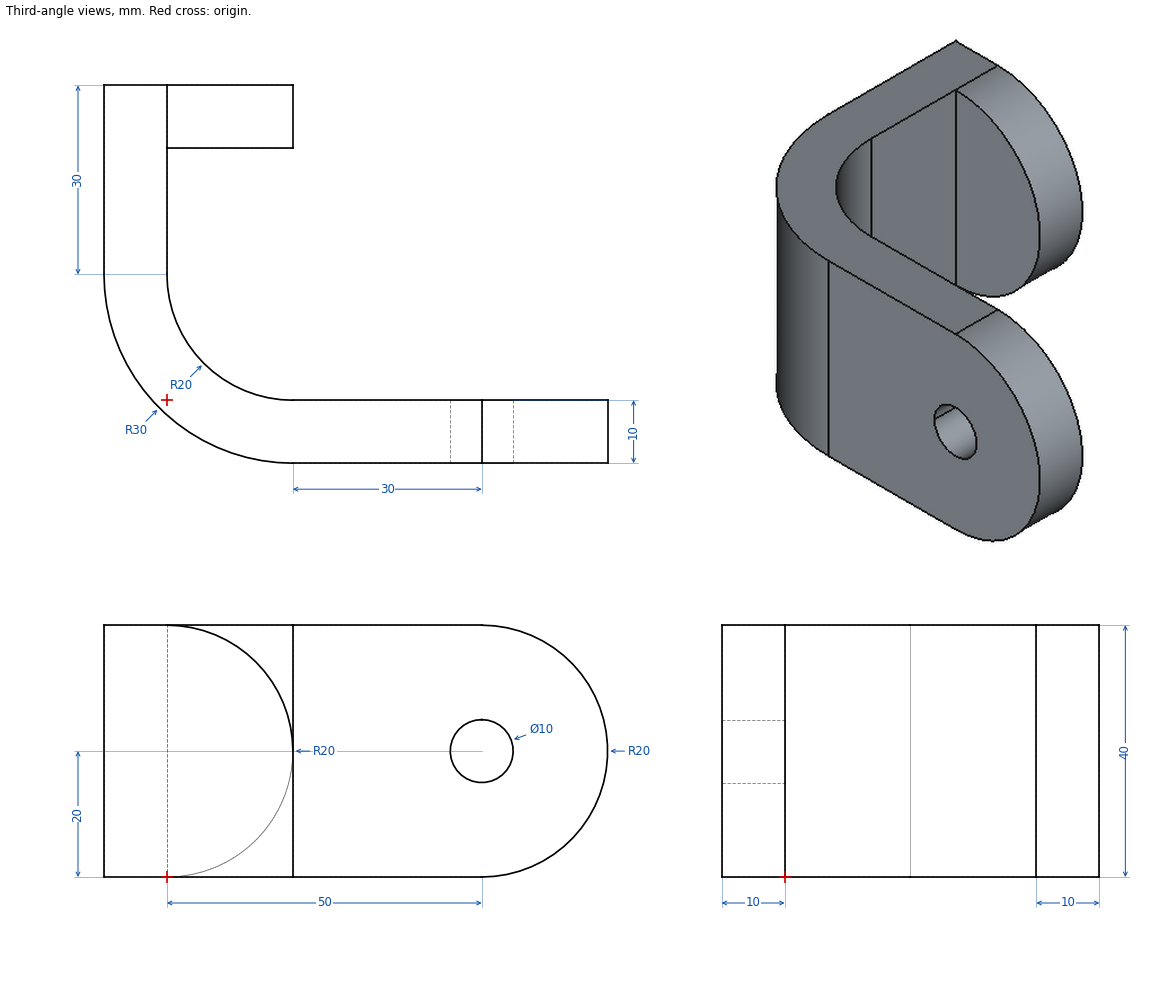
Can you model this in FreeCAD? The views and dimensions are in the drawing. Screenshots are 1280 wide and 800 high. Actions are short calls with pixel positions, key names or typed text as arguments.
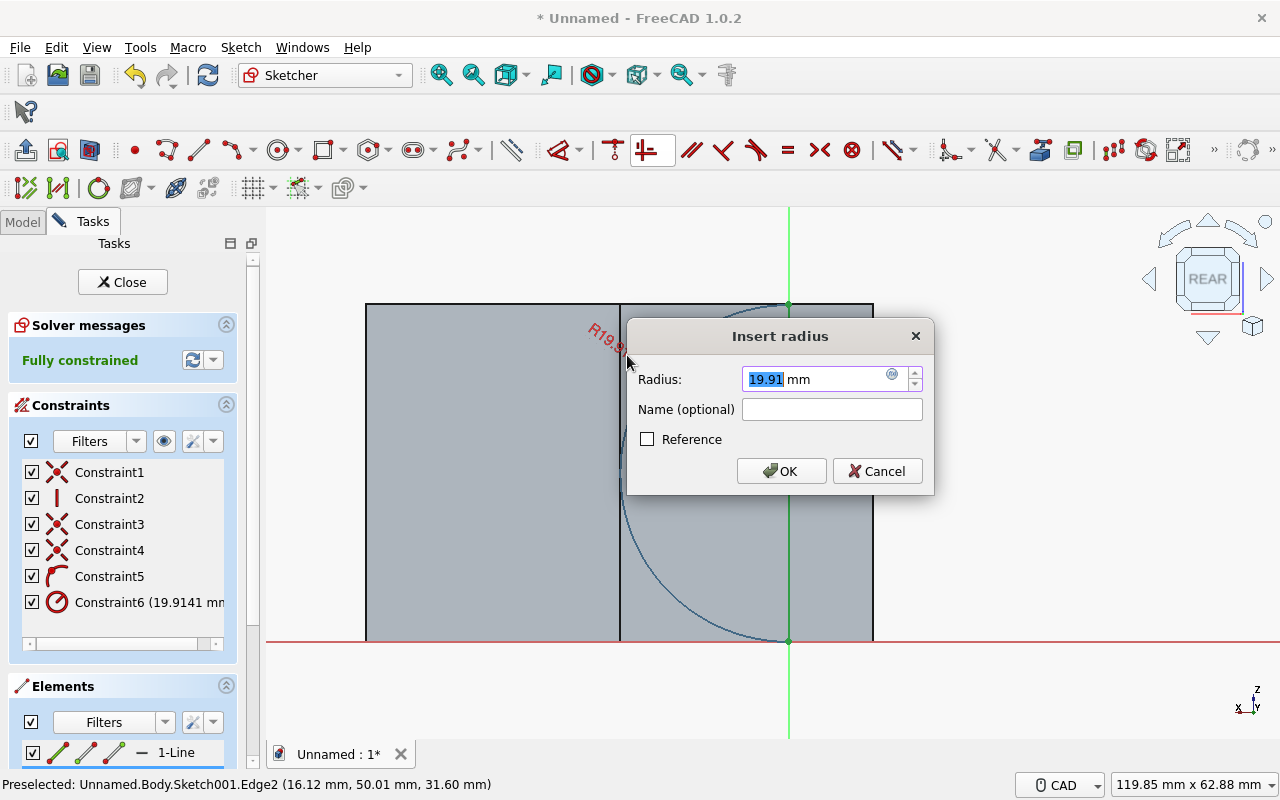
text(20)
key(Return)
key(Escape)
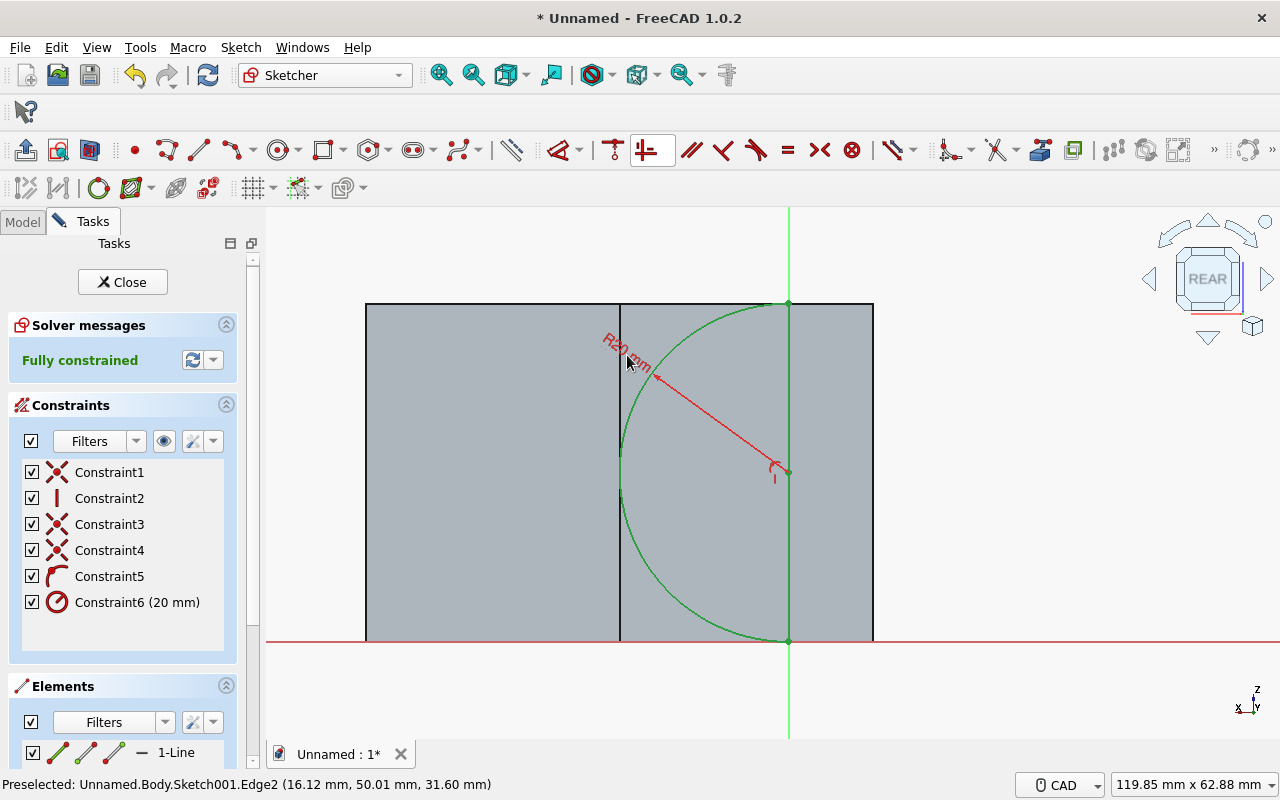
click(123, 282)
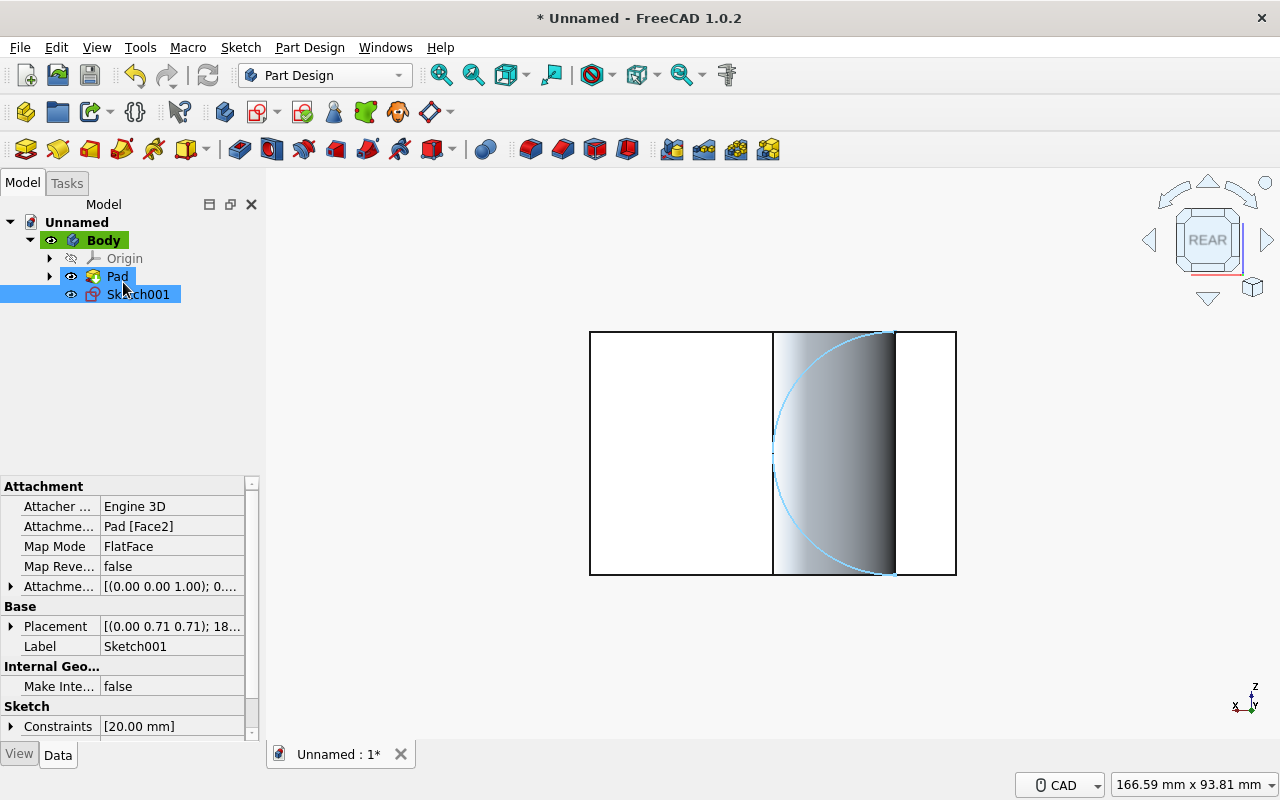
click(26, 150)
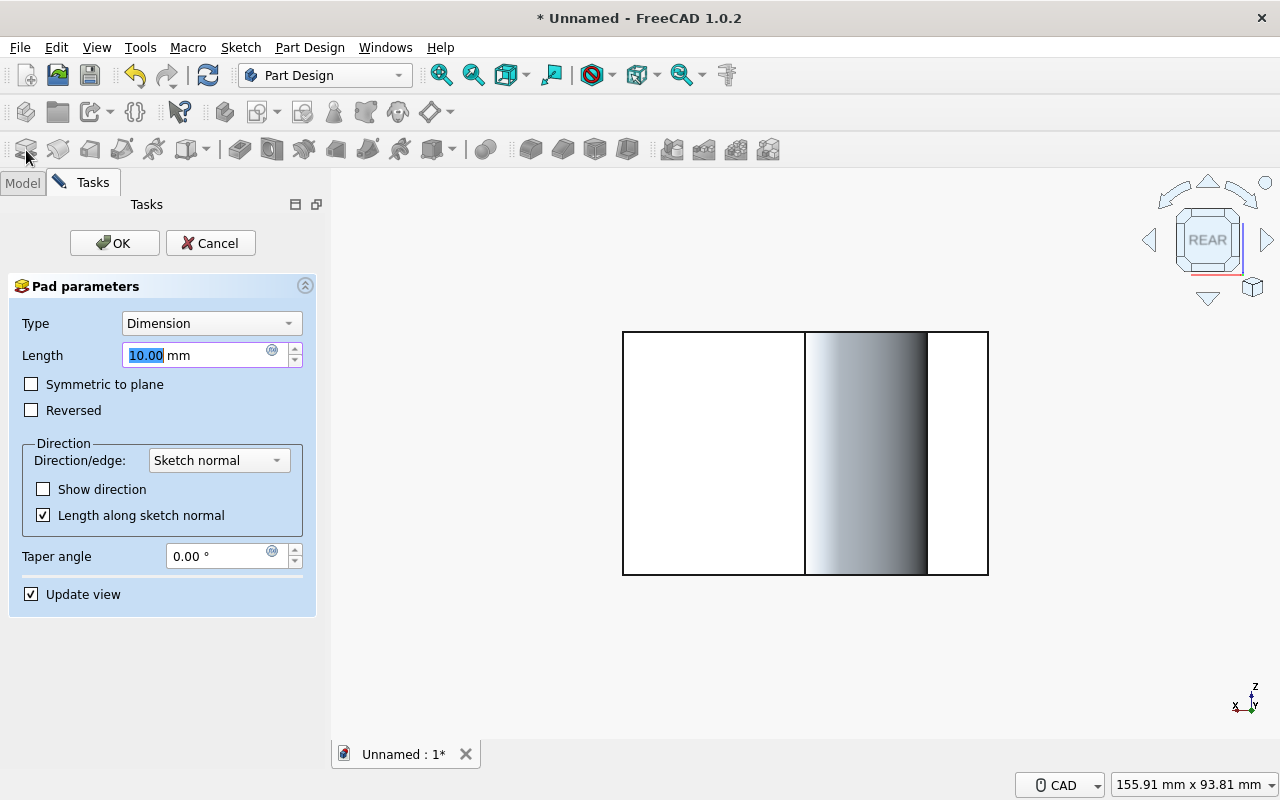
text(10)
key(Tab)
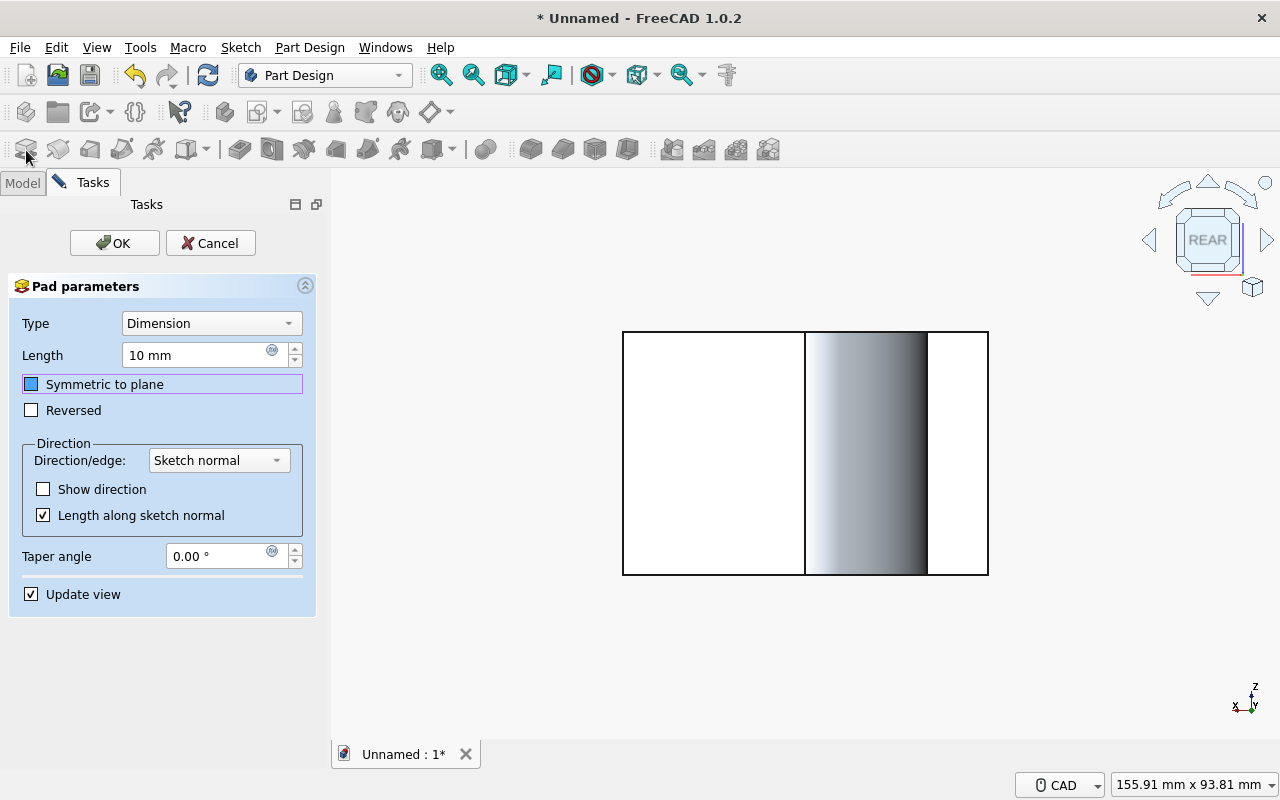
click(30, 410)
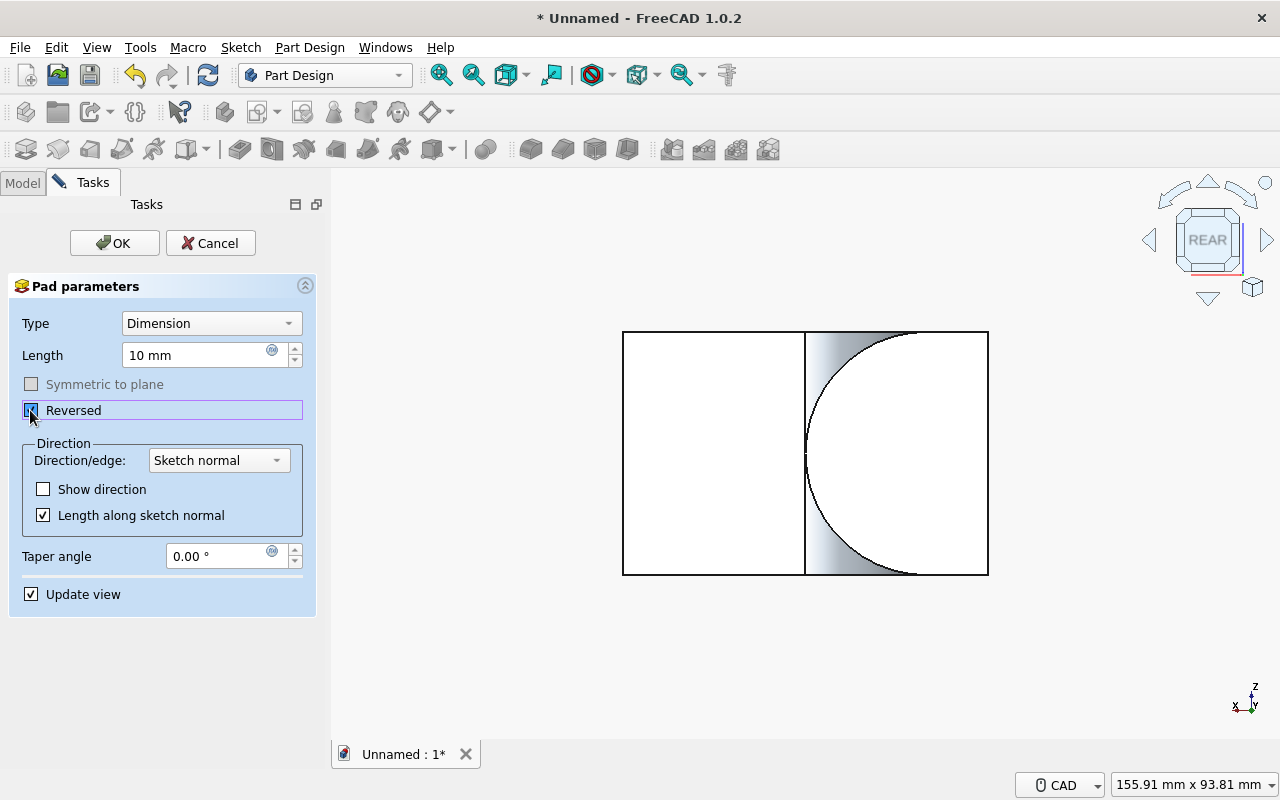
click(115, 243)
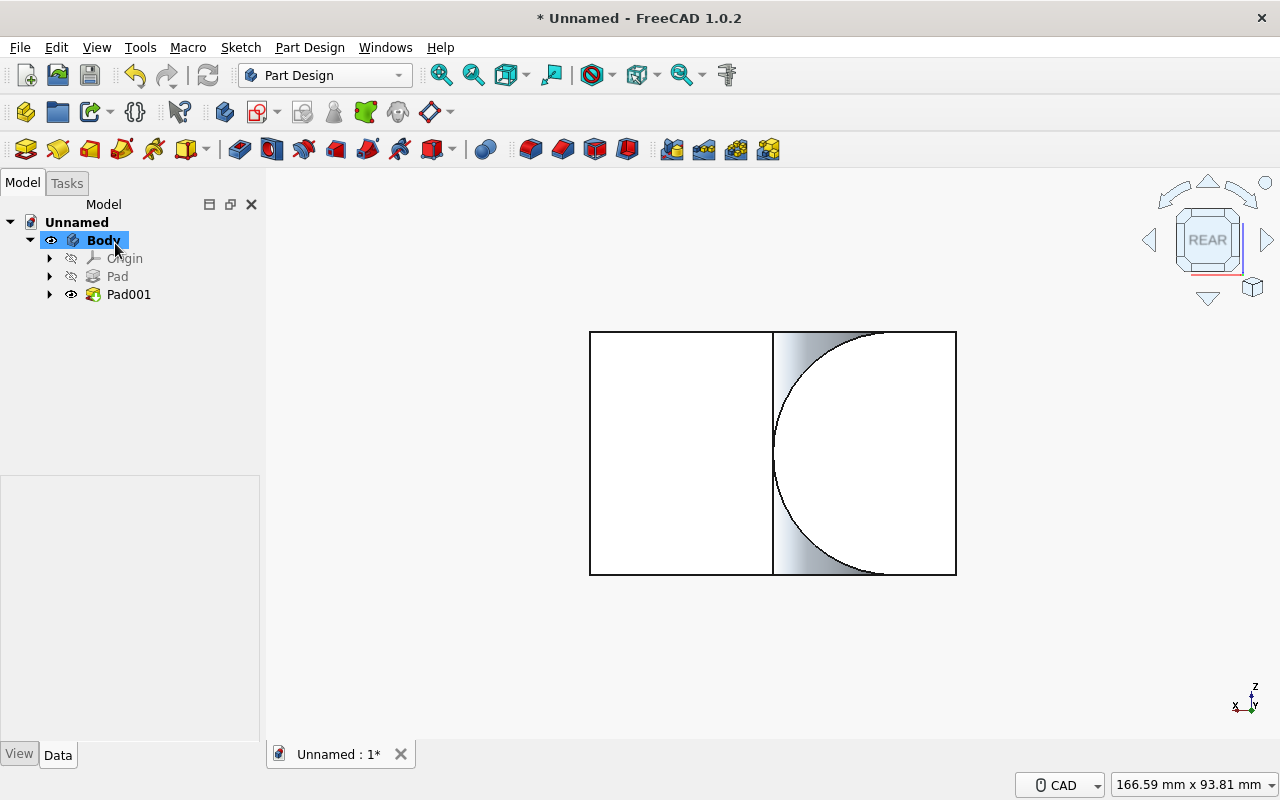
click(442, 76)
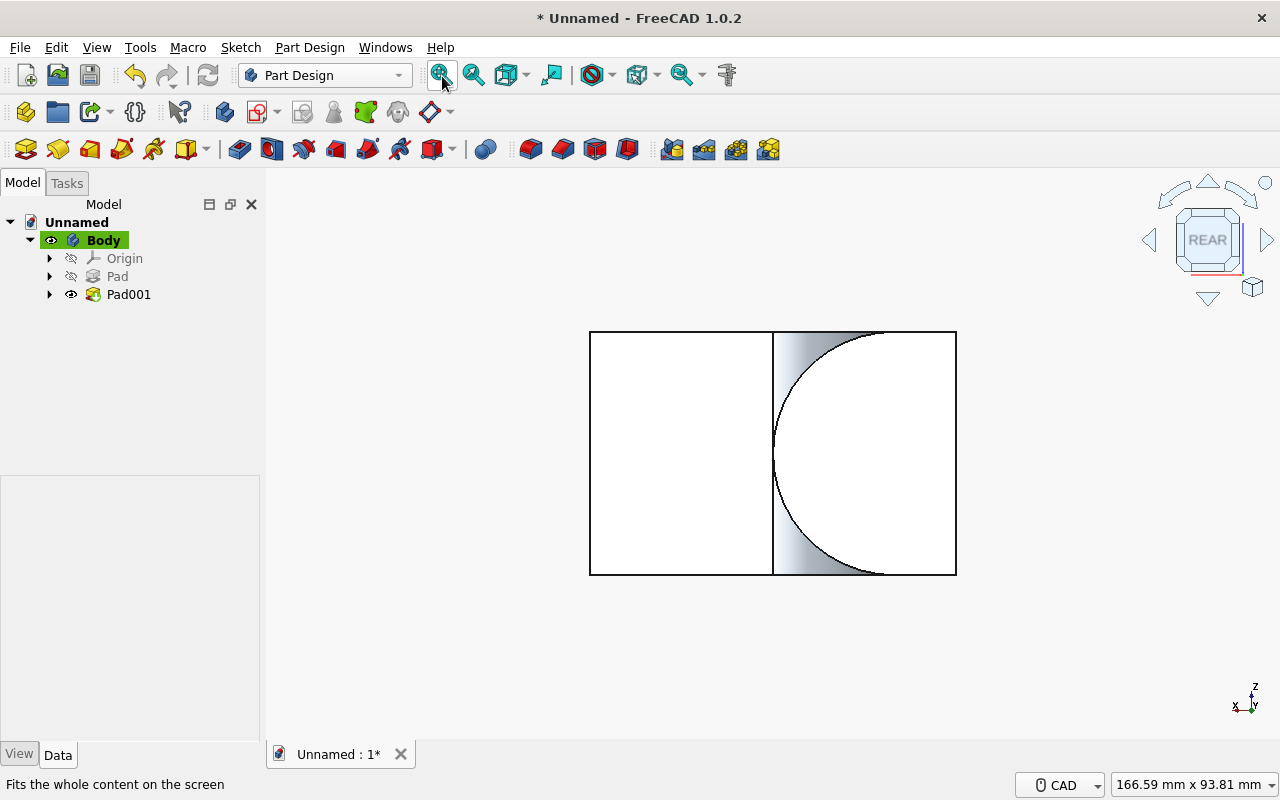
click(682, 452)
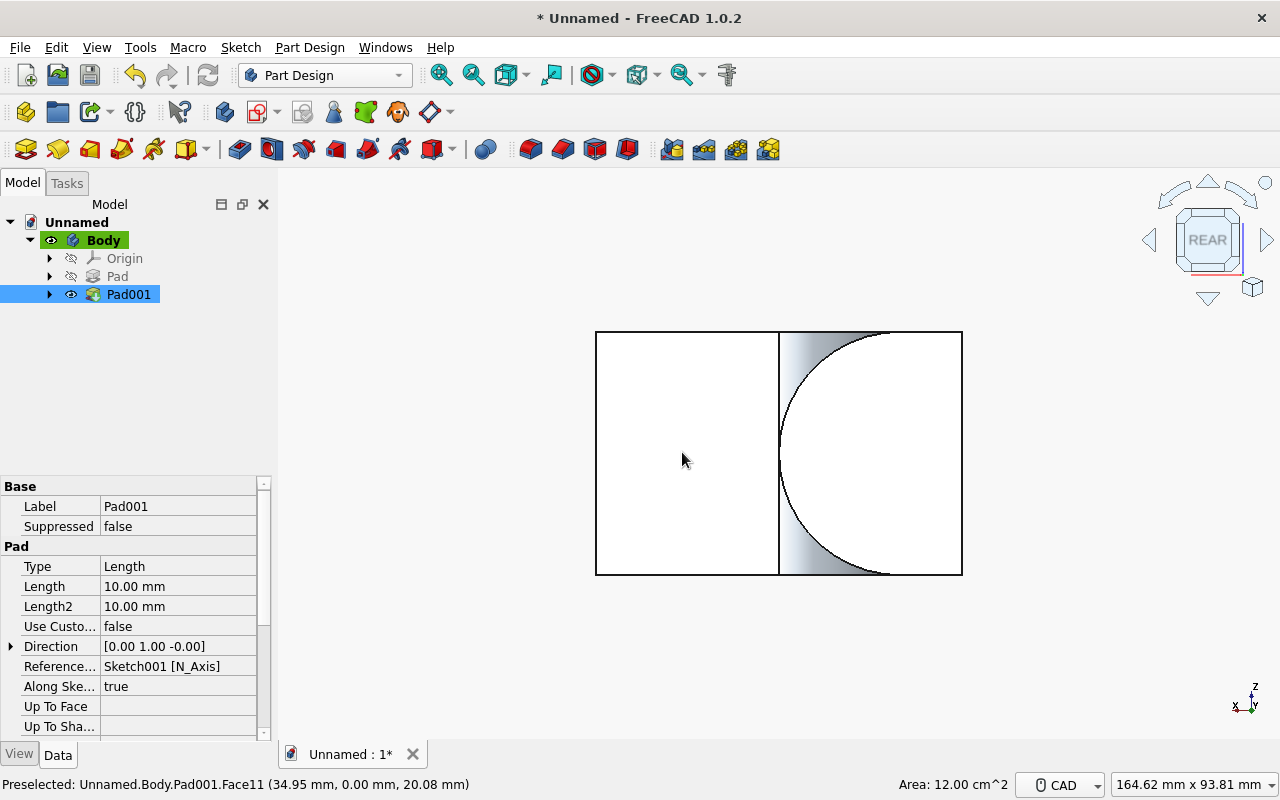
click(258, 112)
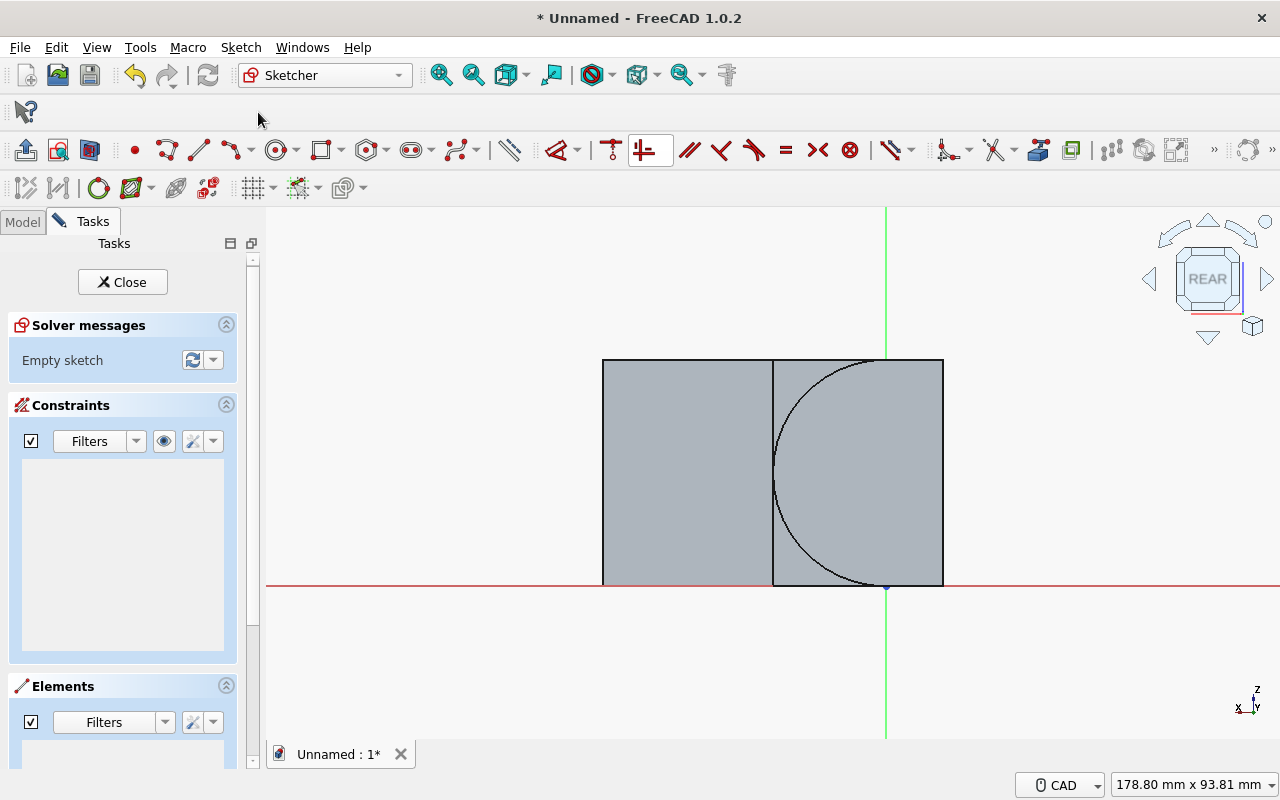
scroll(654, 473, up, 2)